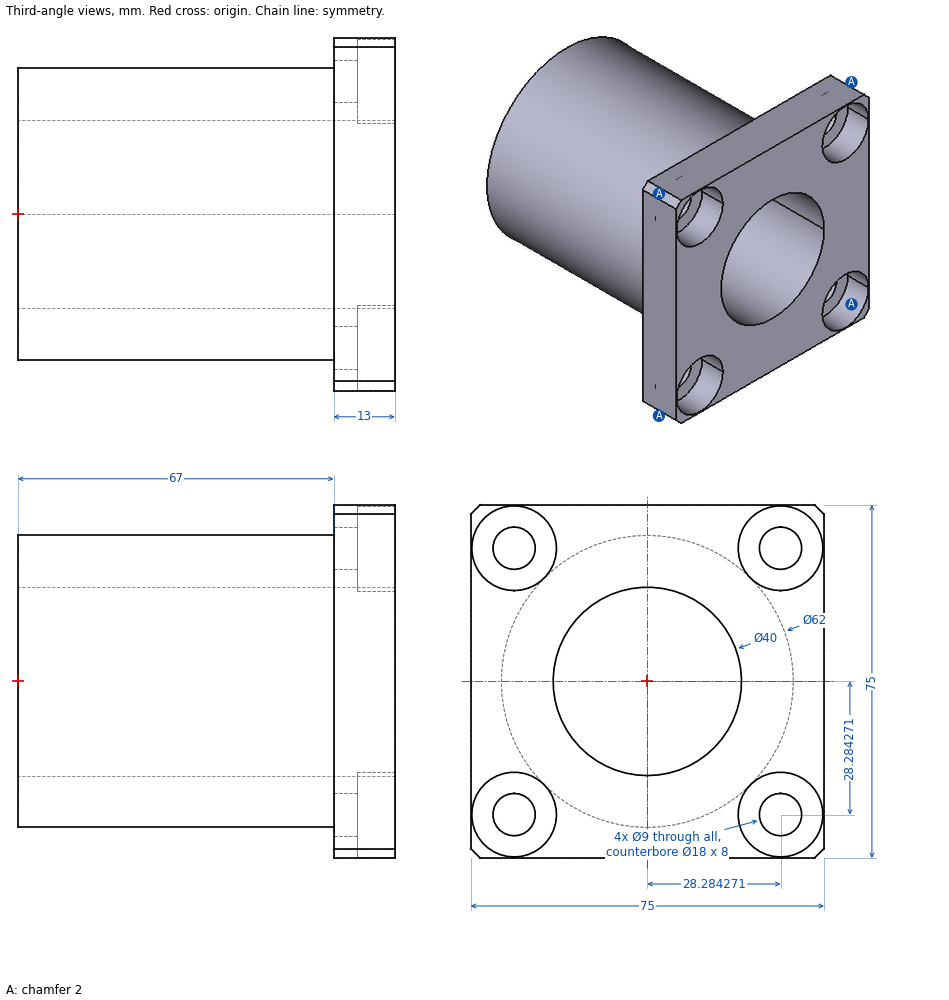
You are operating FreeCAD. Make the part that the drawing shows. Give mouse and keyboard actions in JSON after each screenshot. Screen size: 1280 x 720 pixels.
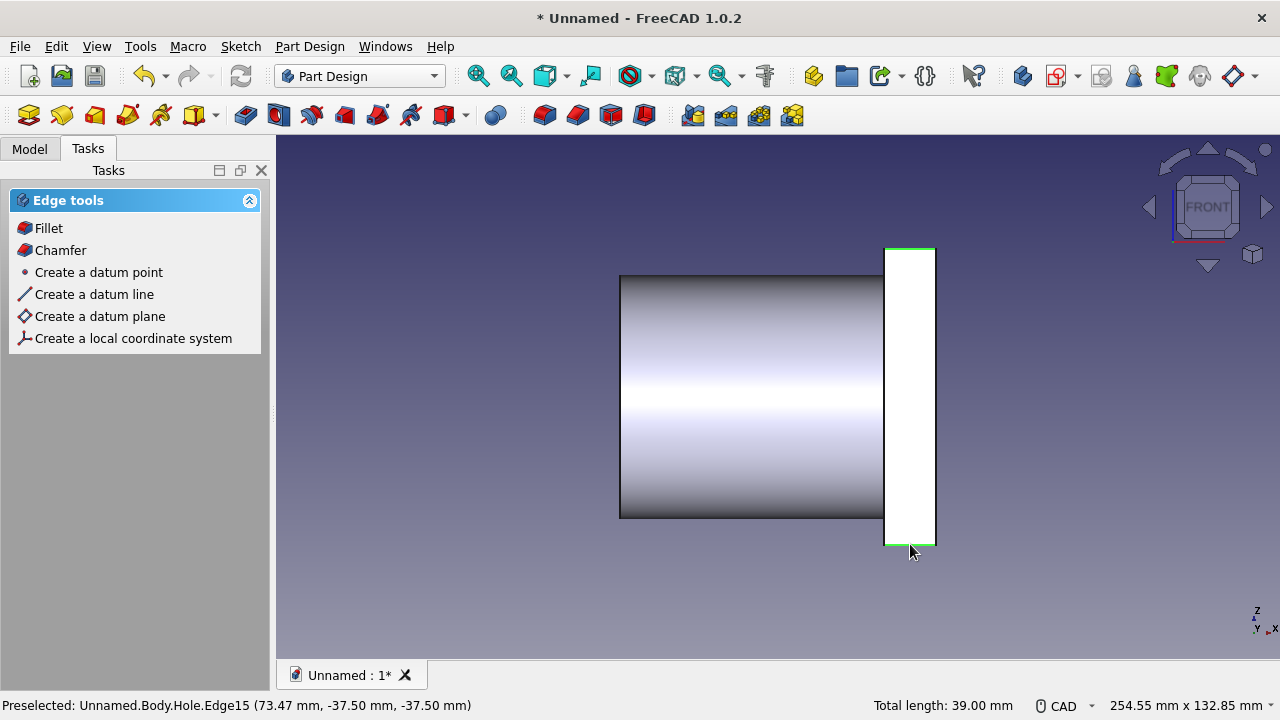
{"action": "key", "text": "3"}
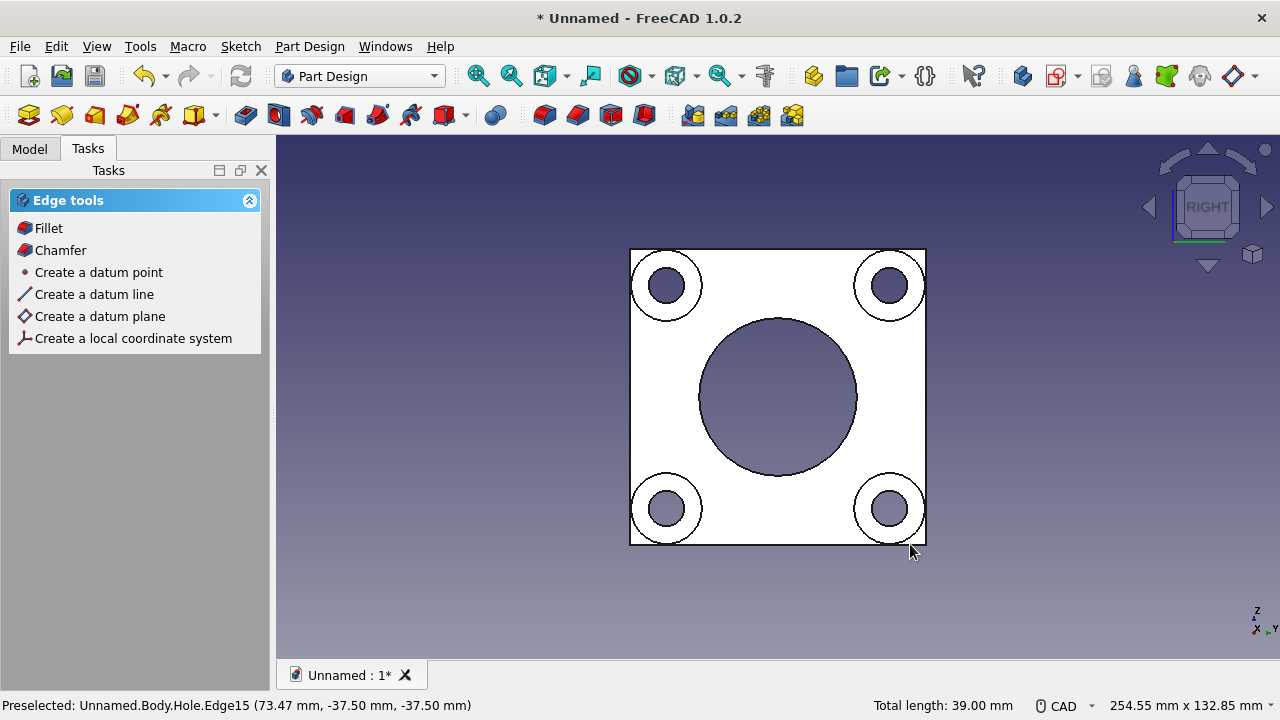
{"action": "key", "text": "5"}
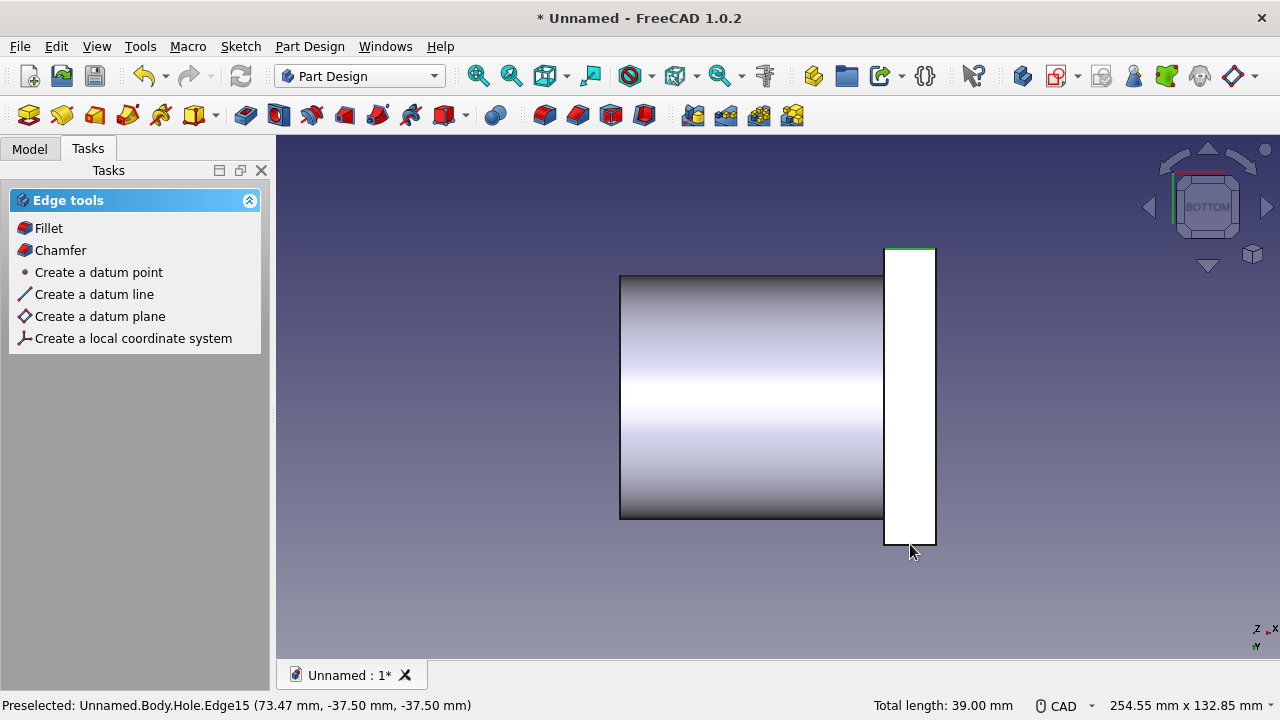
{"action": "left_click", "coordinate": [910, 544], "text": "ctrl"}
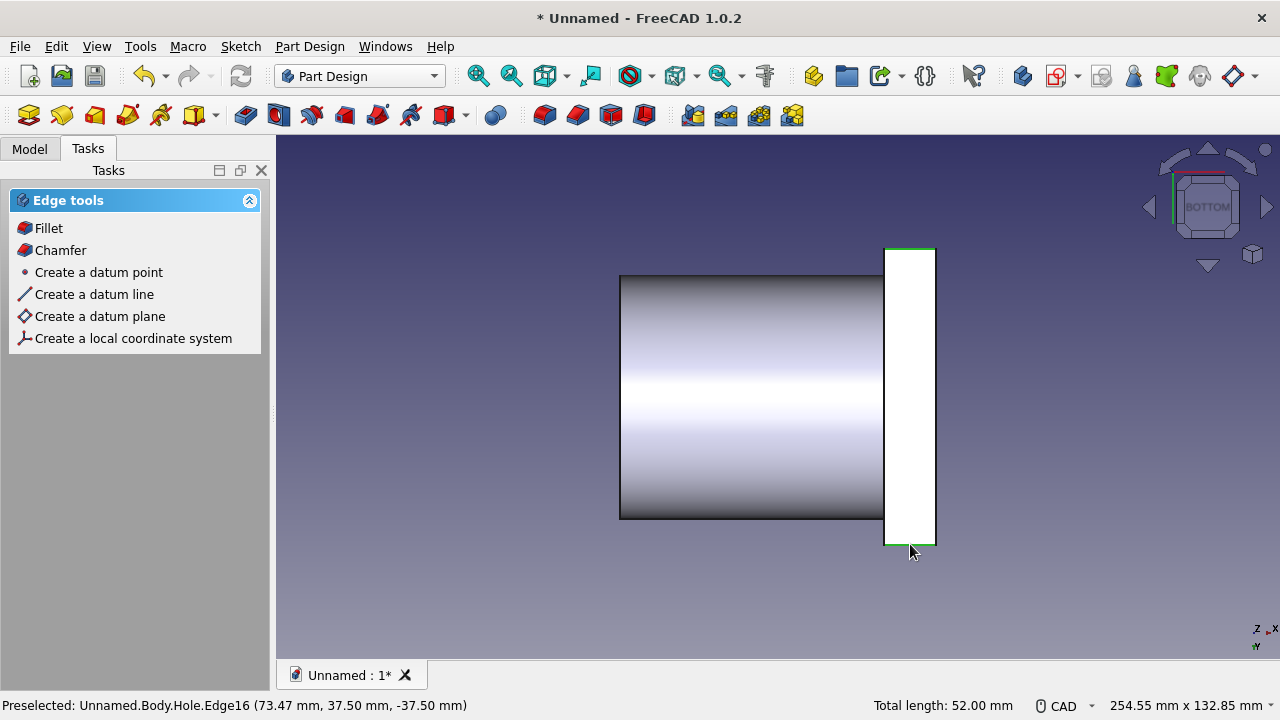
{"action": "left_click", "coordinate": [578, 116]}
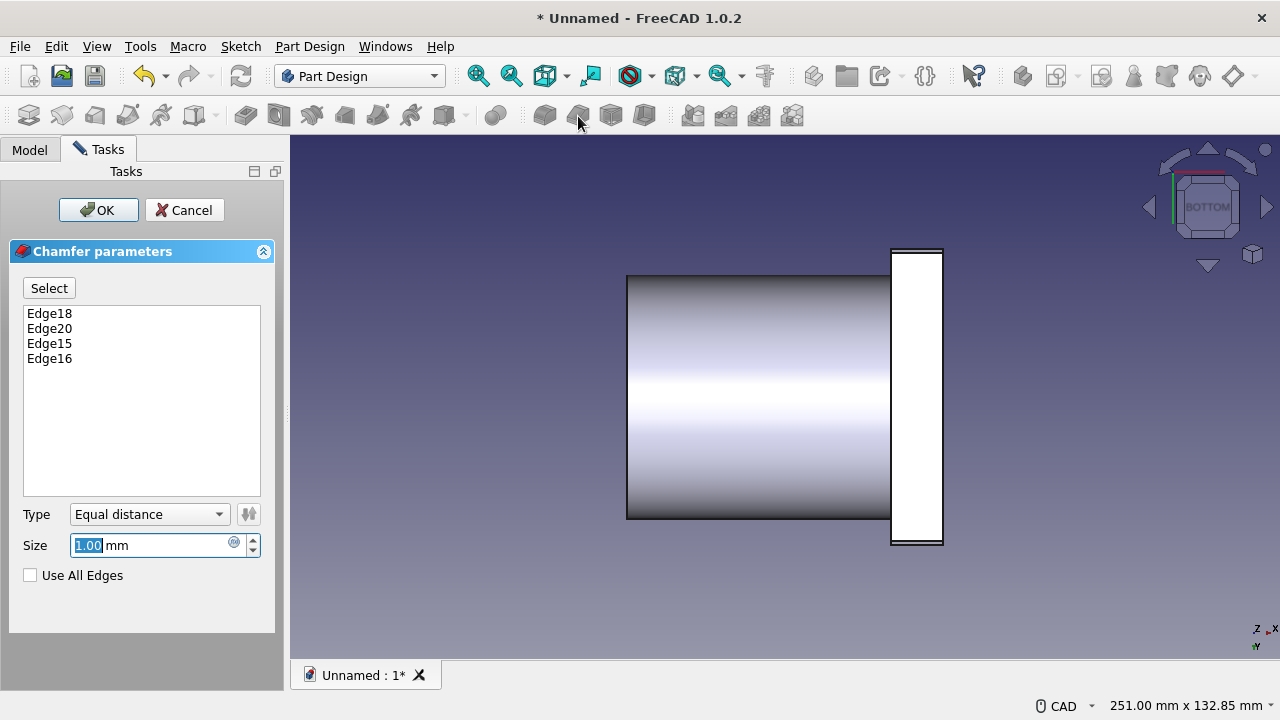
{"action": "type", "text": "2"}
{"action": "key", "text": "Tab"}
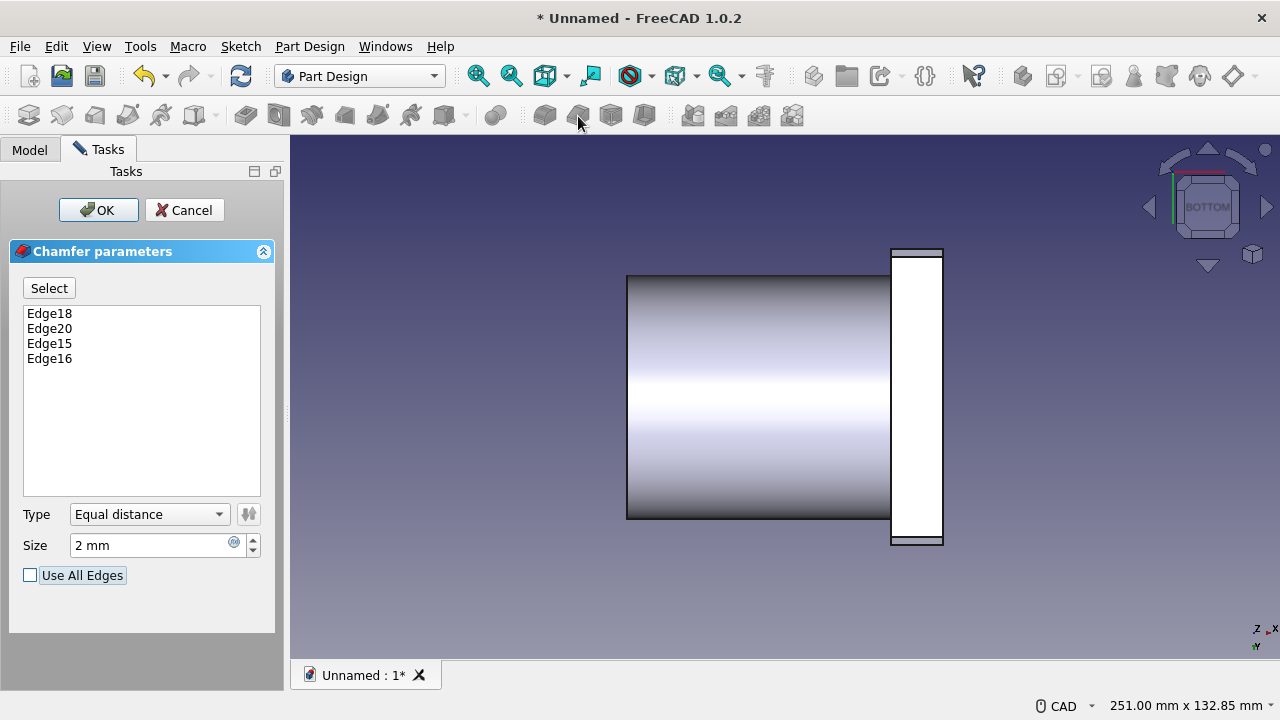
{"action": "left_click", "coordinate": [99, 210]}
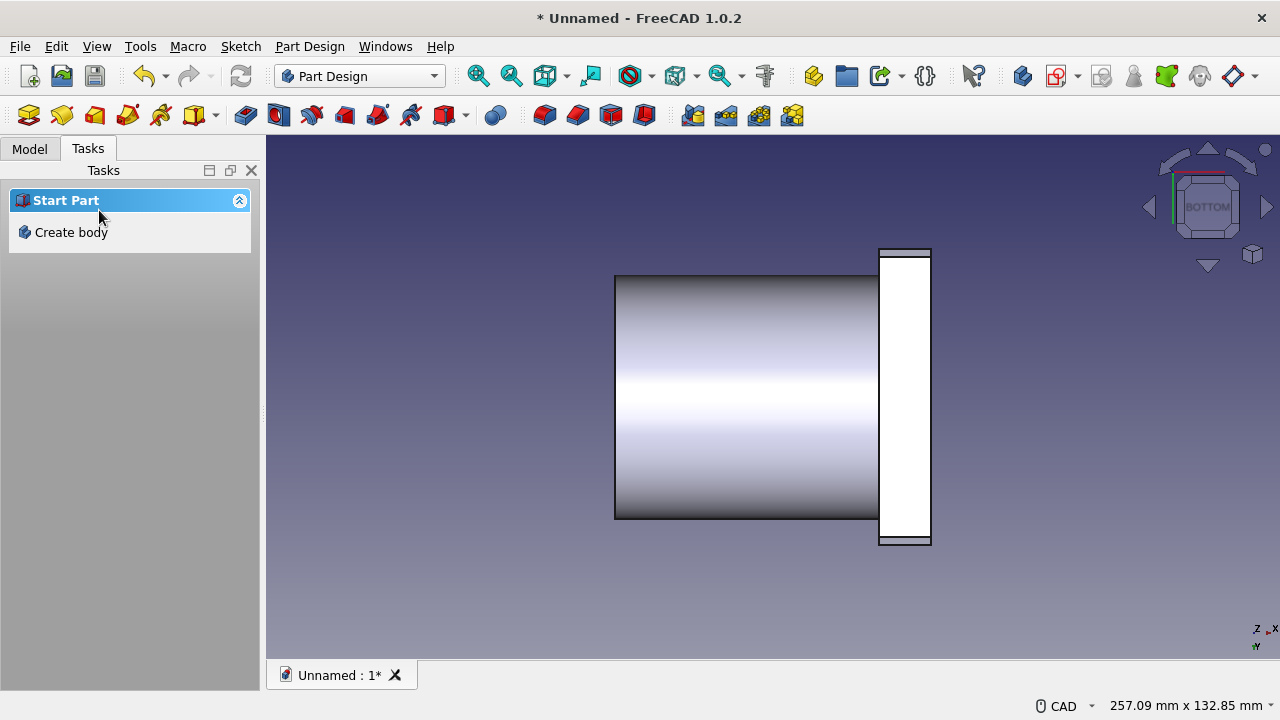
{"action": "key", "text": "0"}